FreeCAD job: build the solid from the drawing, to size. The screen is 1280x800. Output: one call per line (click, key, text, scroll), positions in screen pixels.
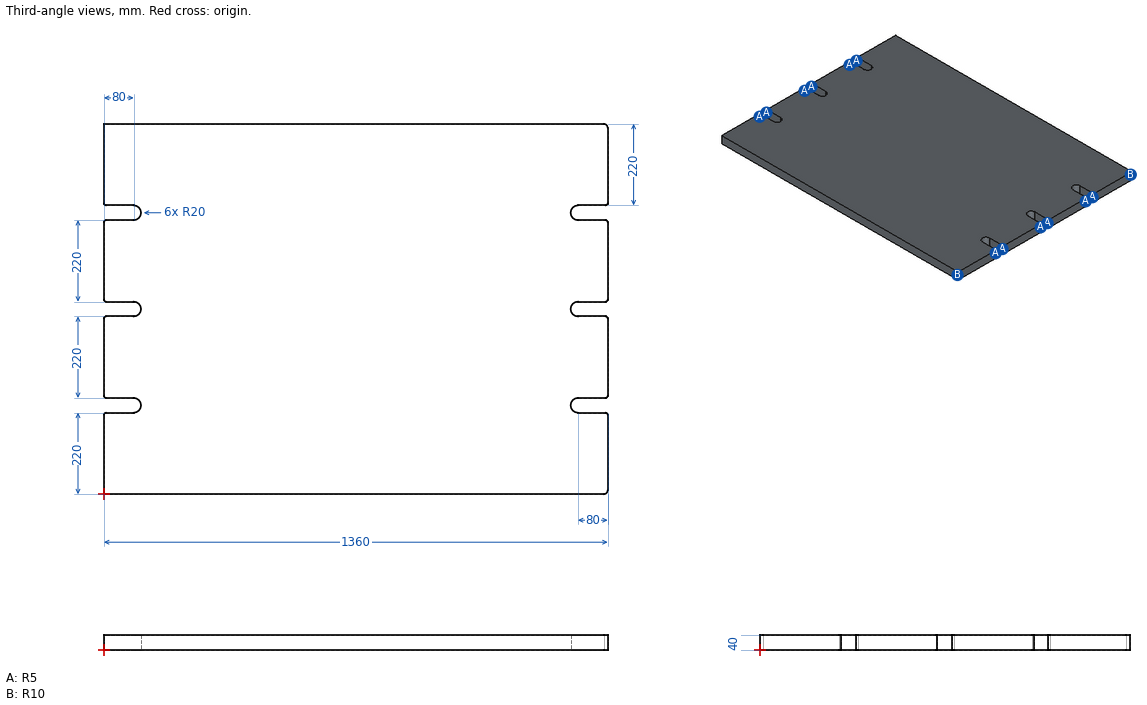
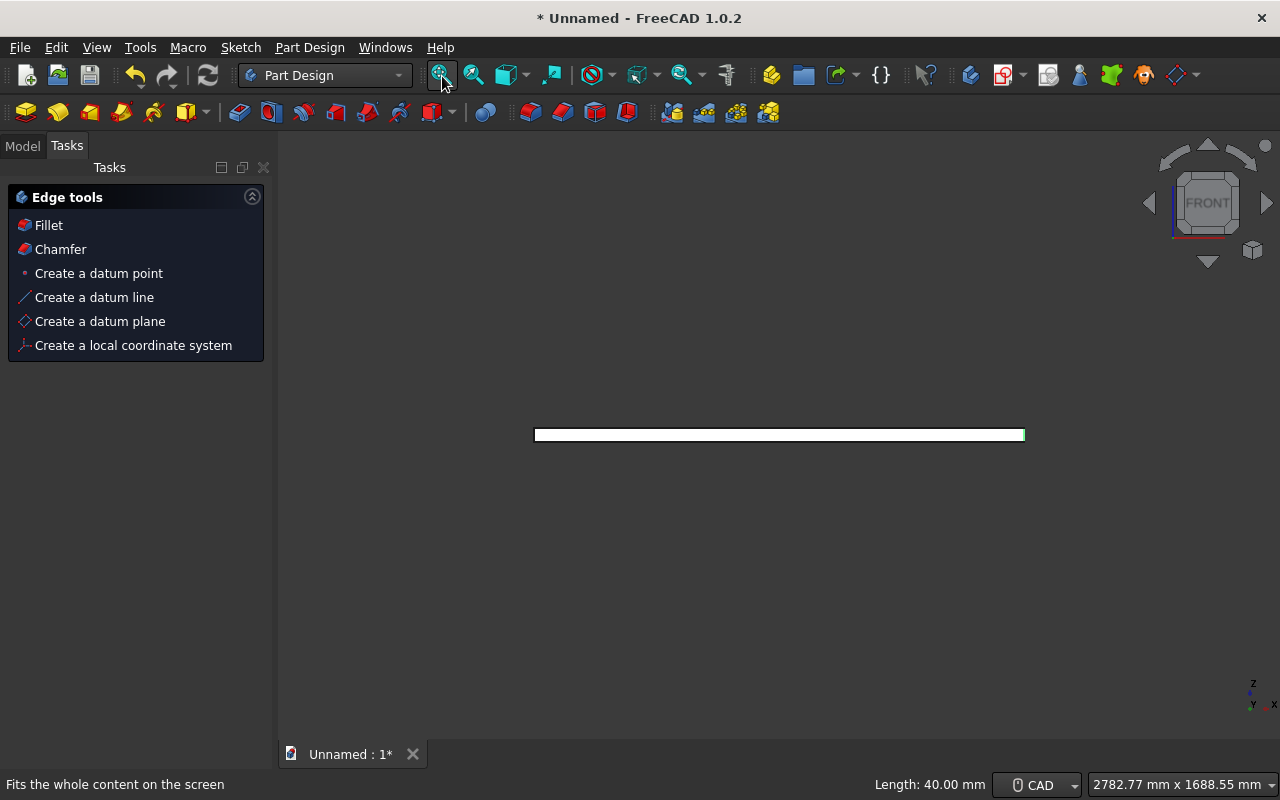
scroll(1024, 434, up, 6)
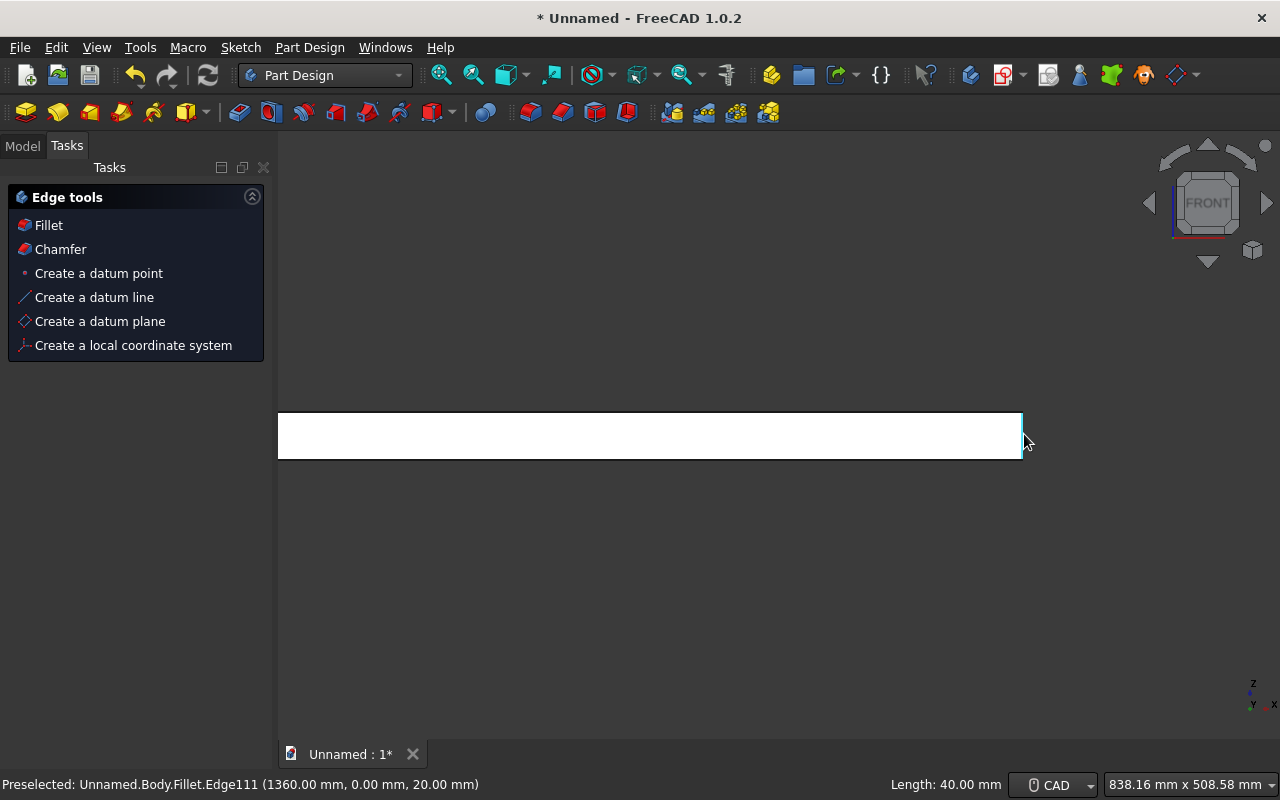
click(442, 76)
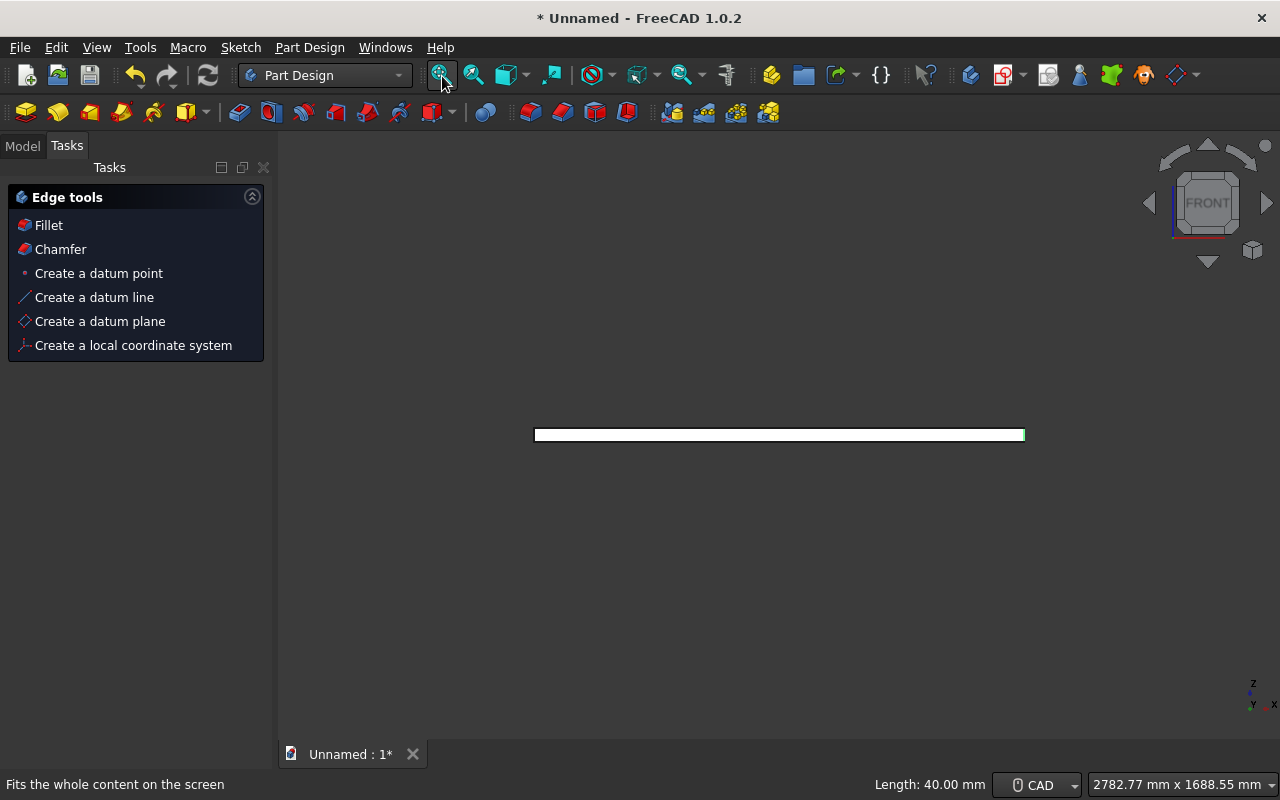
key(3)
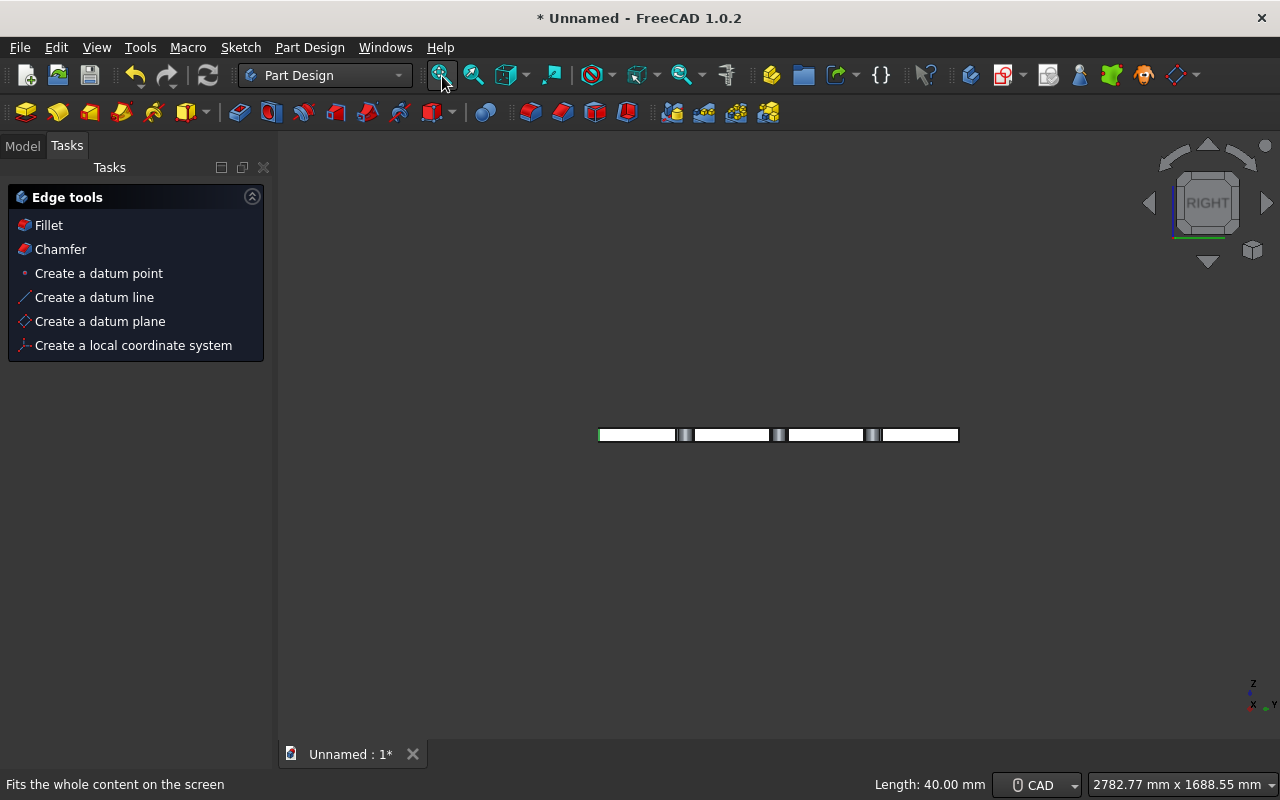
click(442, 76)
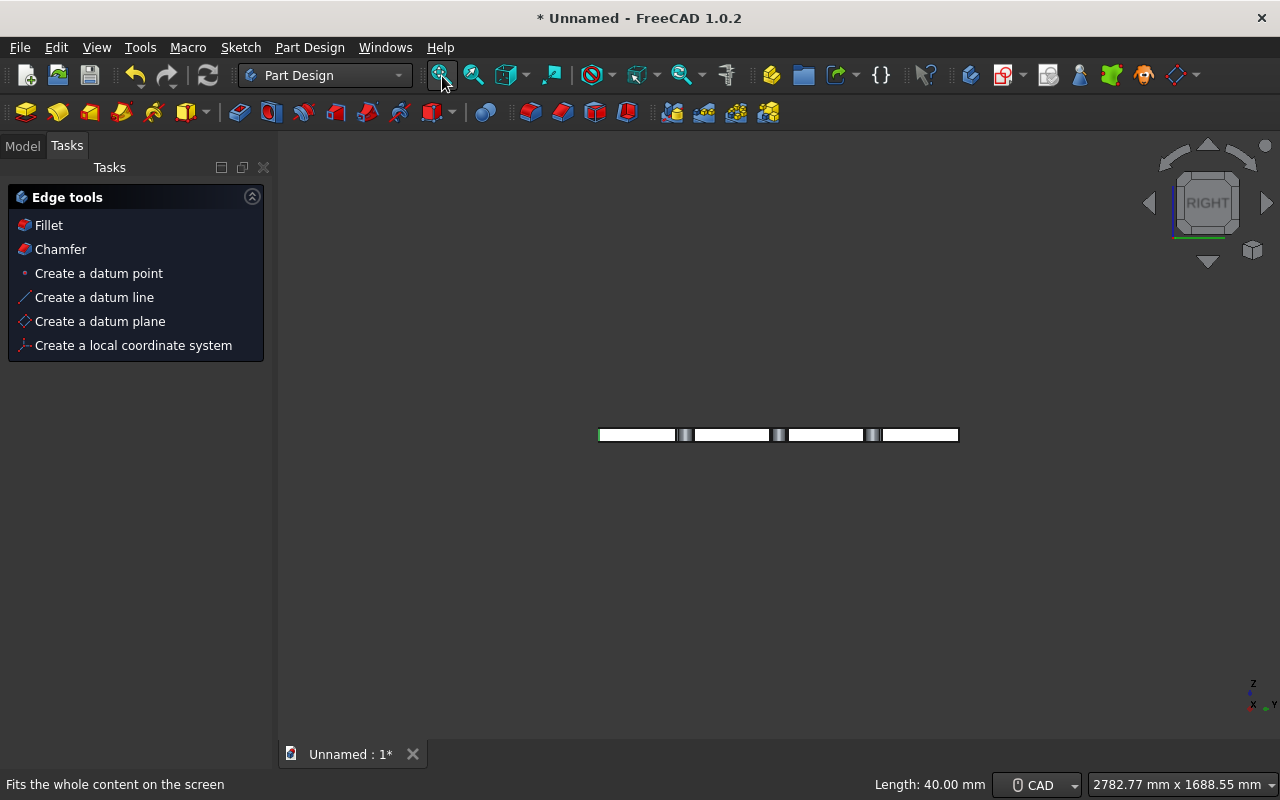
click(959, 434, ctrl)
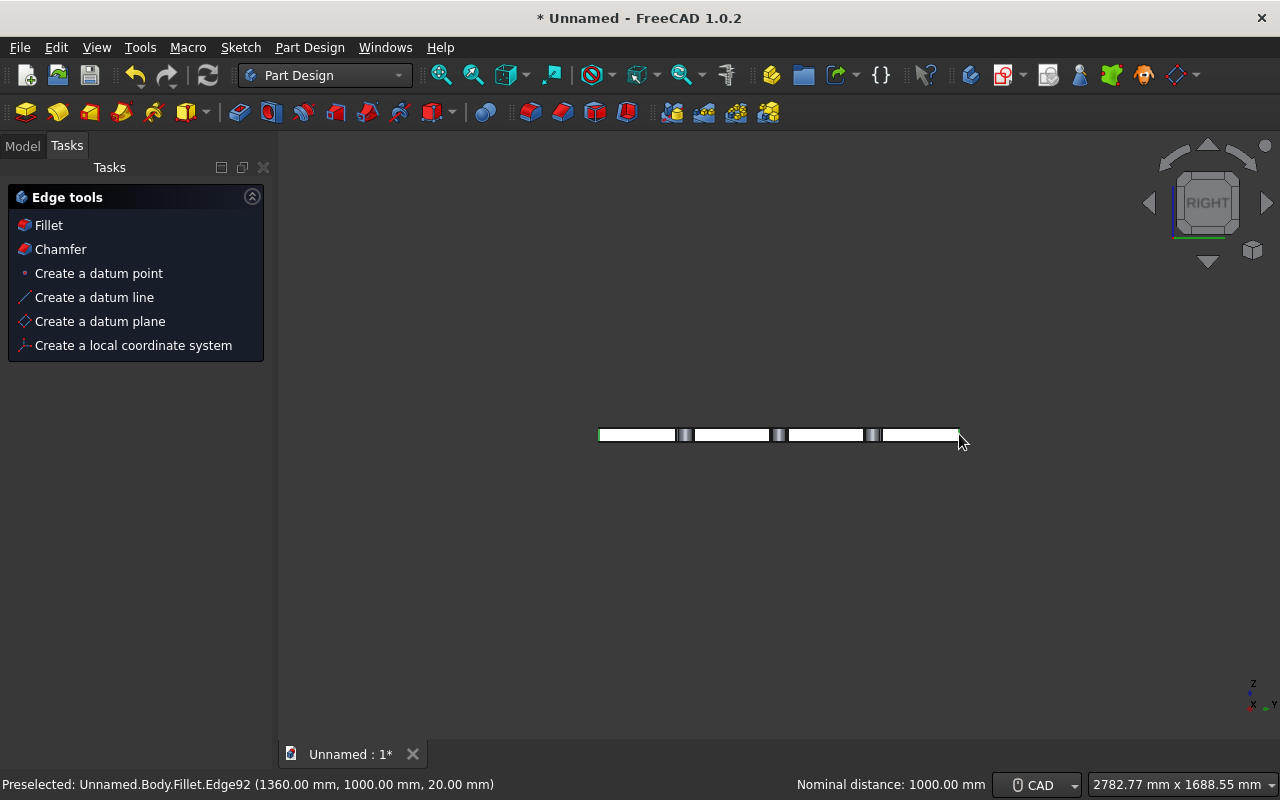
click(532, 112)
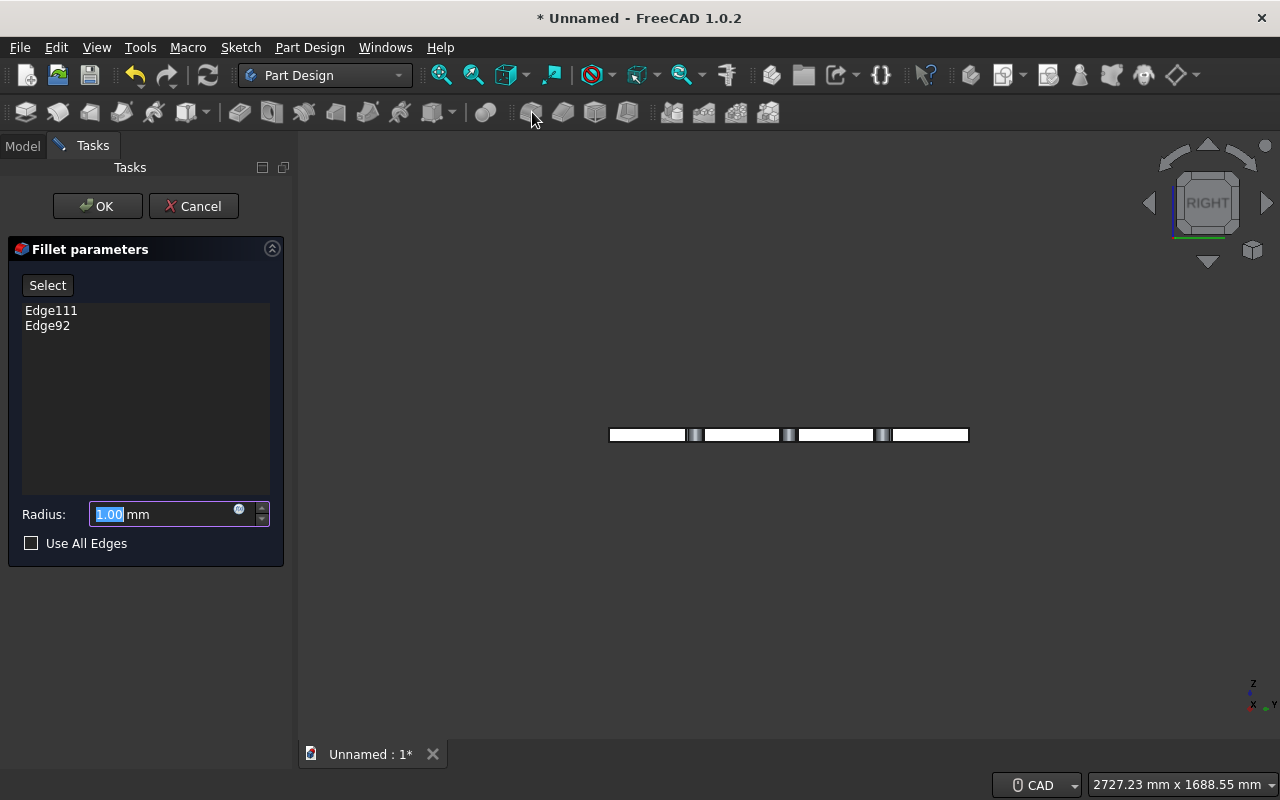
text(10)
key(Tab)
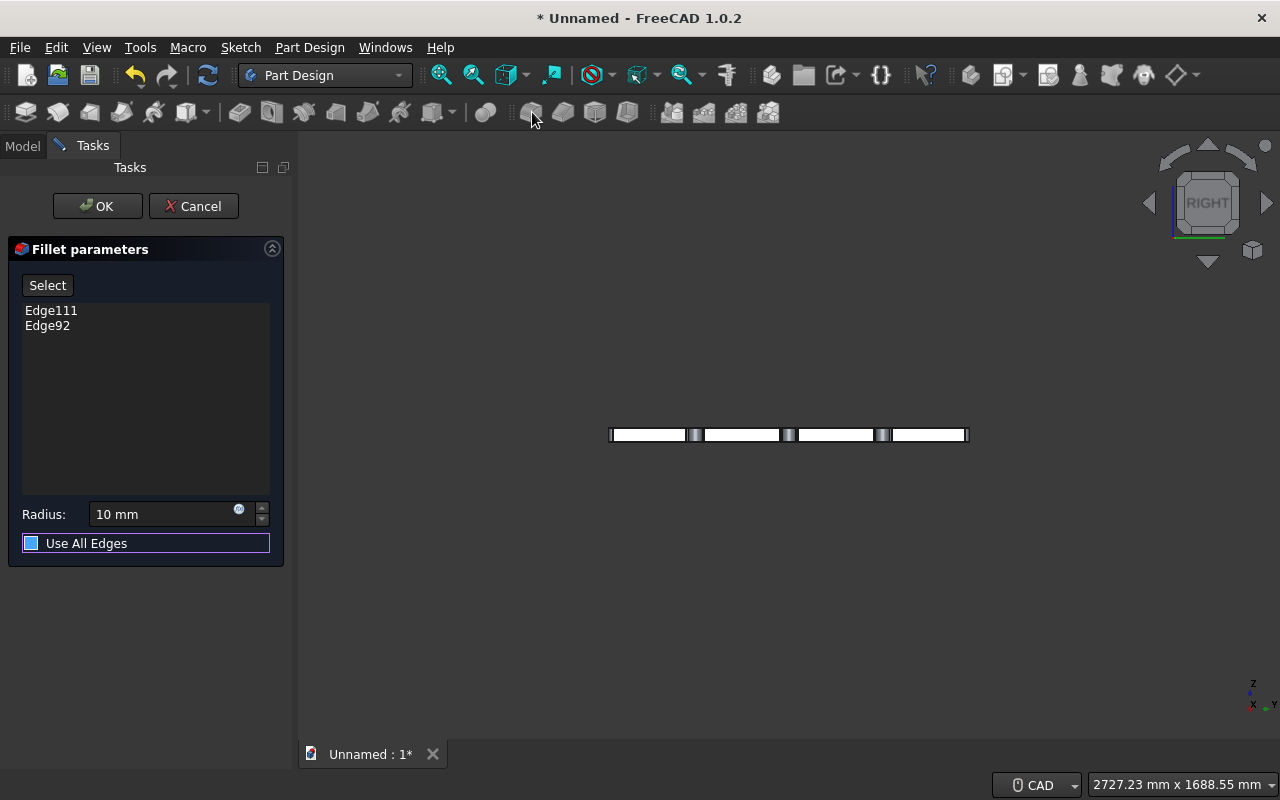
click(98, 206)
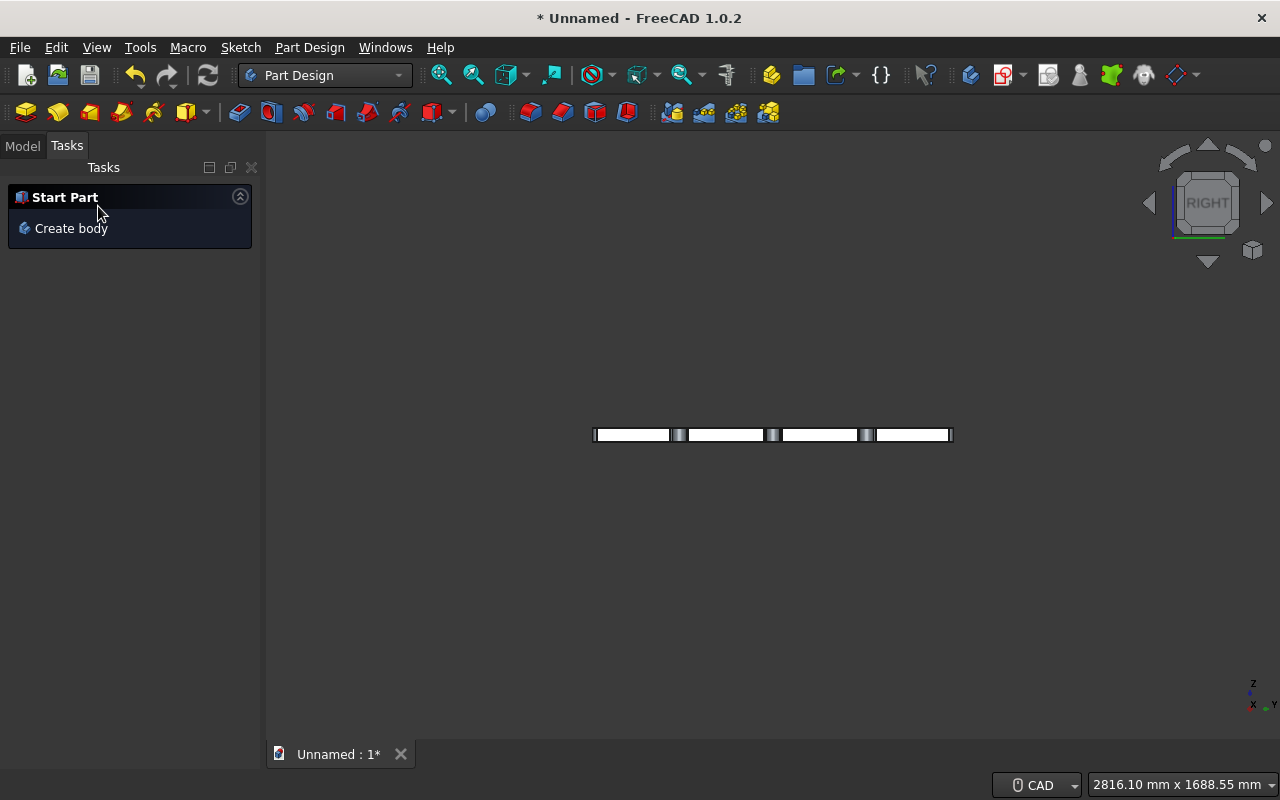
key(0)